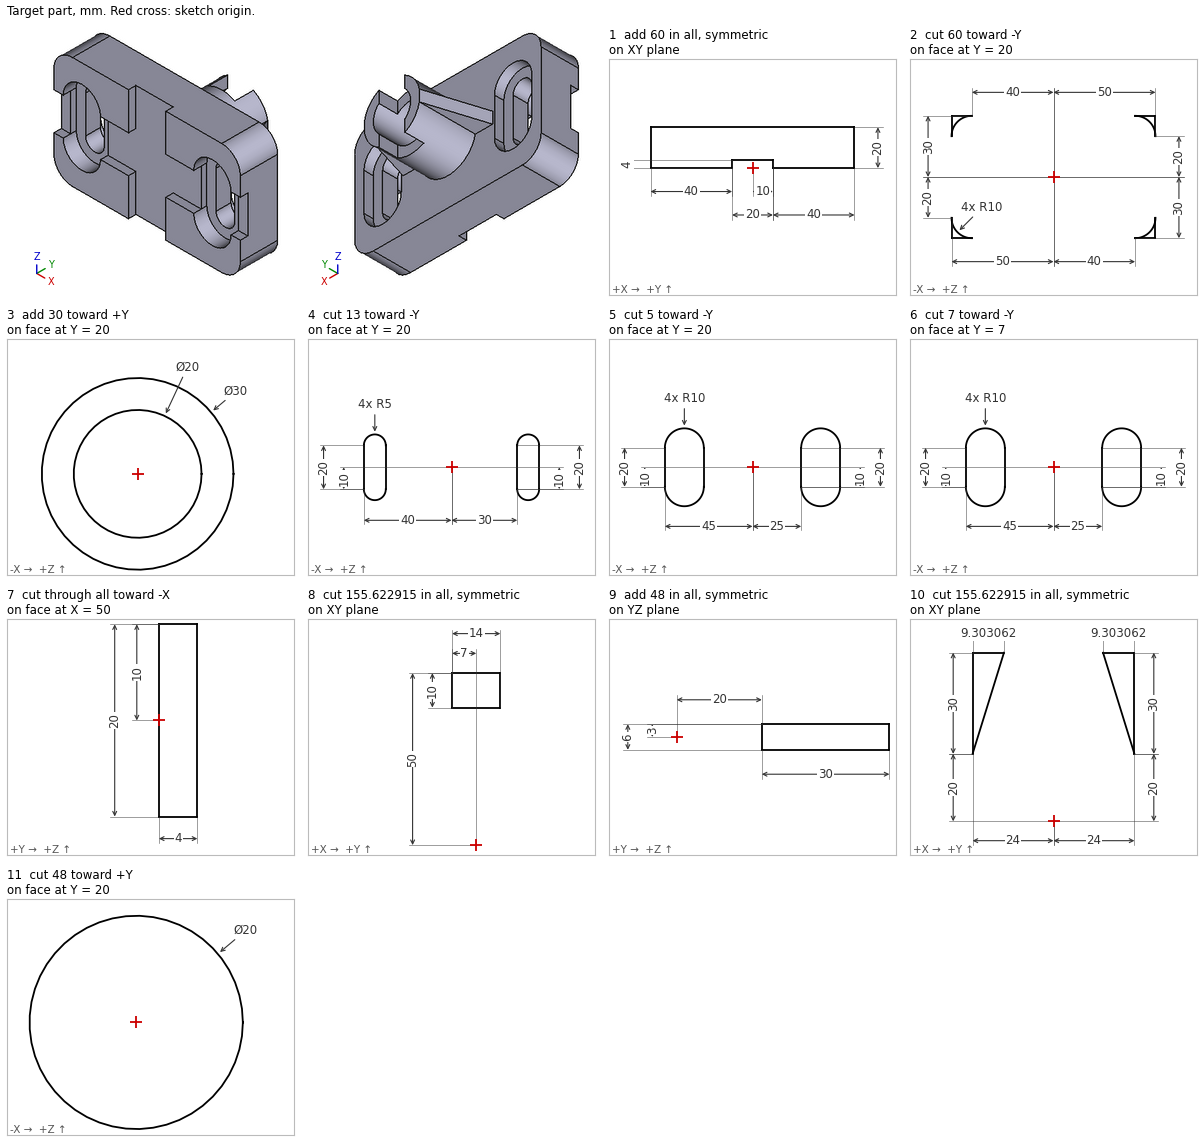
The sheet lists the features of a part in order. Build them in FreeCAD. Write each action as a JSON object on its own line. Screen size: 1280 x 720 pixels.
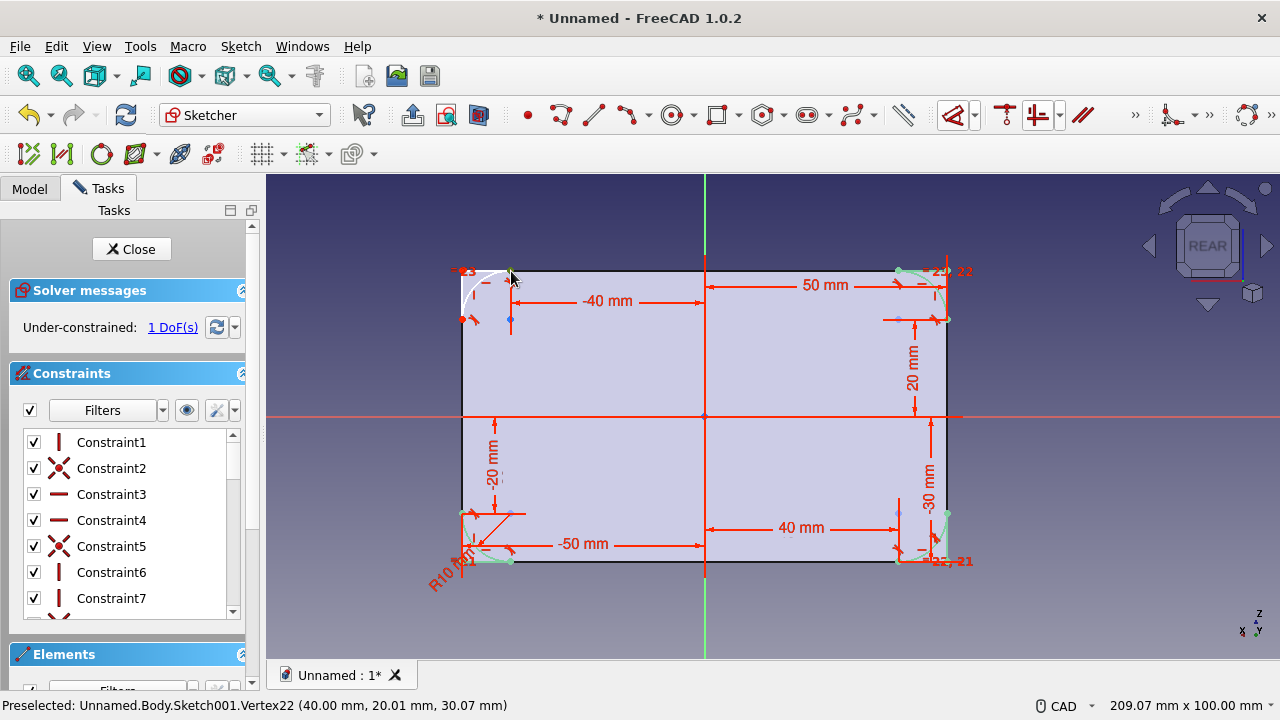
{"action": "left_click", "coordinate": [974, 116]}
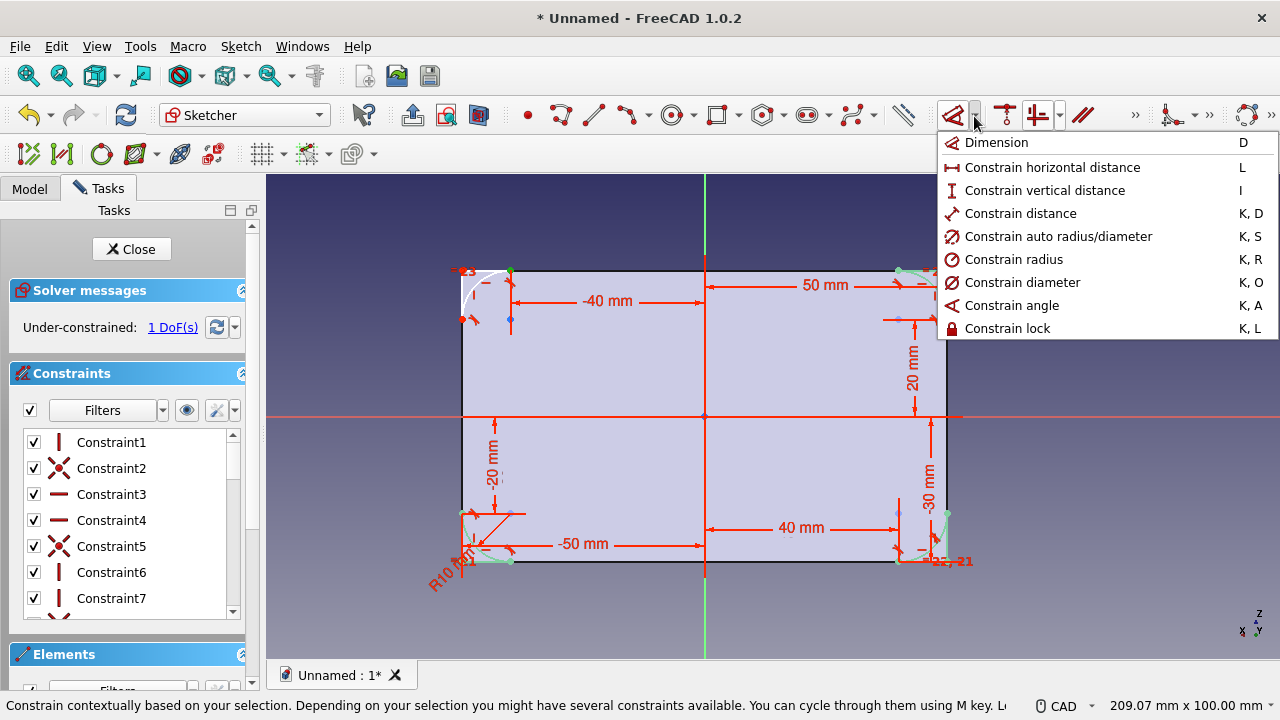
{"action": "left_click", "coordinate": [1108, 190]}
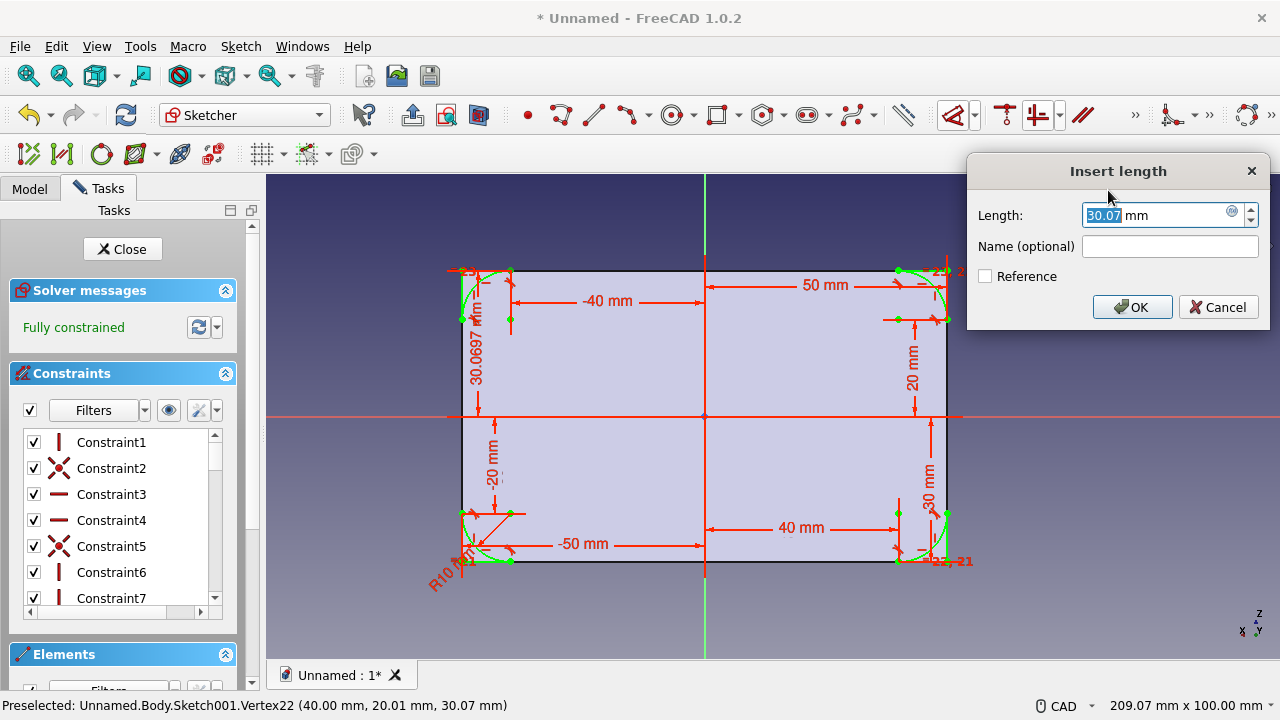
{"action": "type", "text": "30"}
{"action": "key", "text": "Return"}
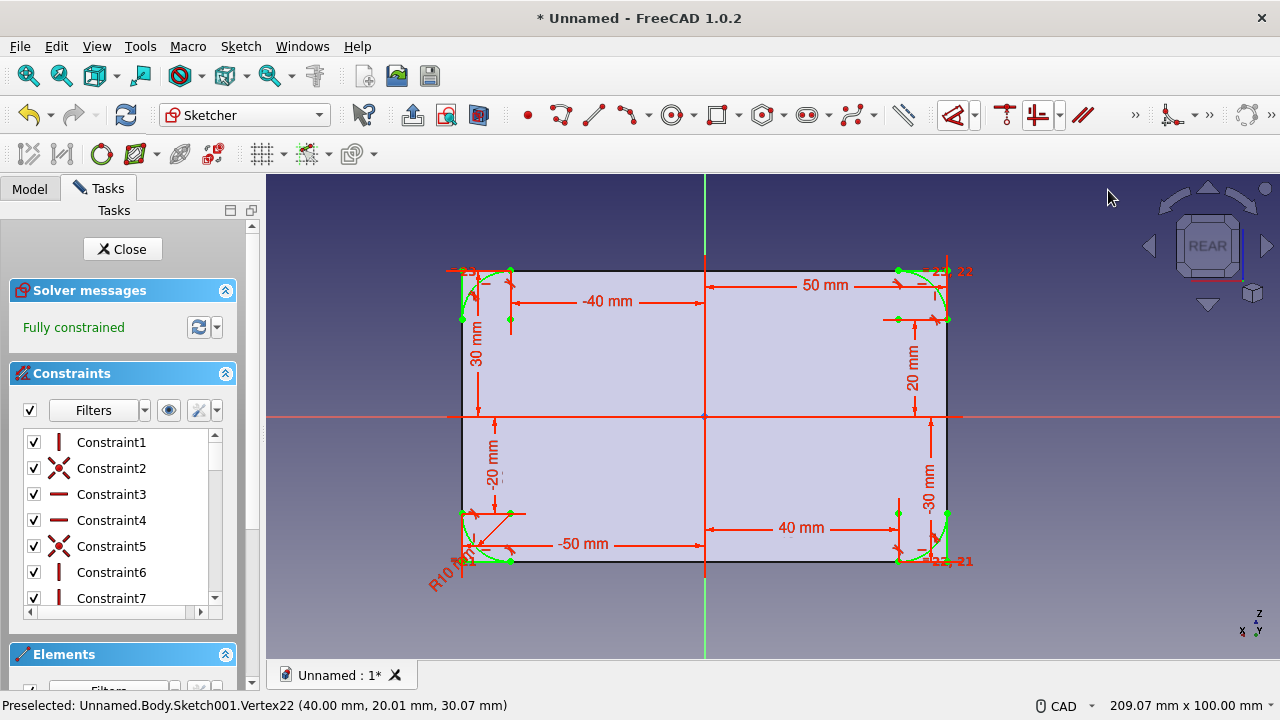
{"action": "left_click", "coordinate": [123, 249]}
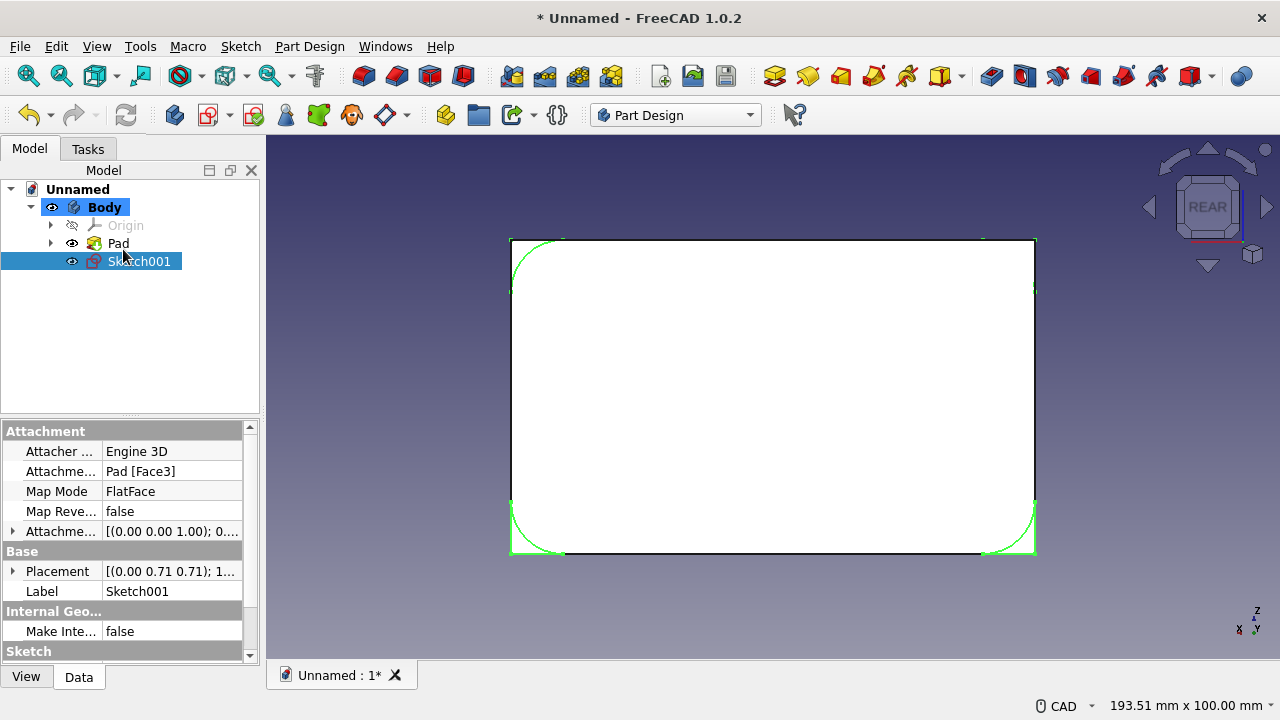
{"action": "left_click", "coordinate": [992, 76]}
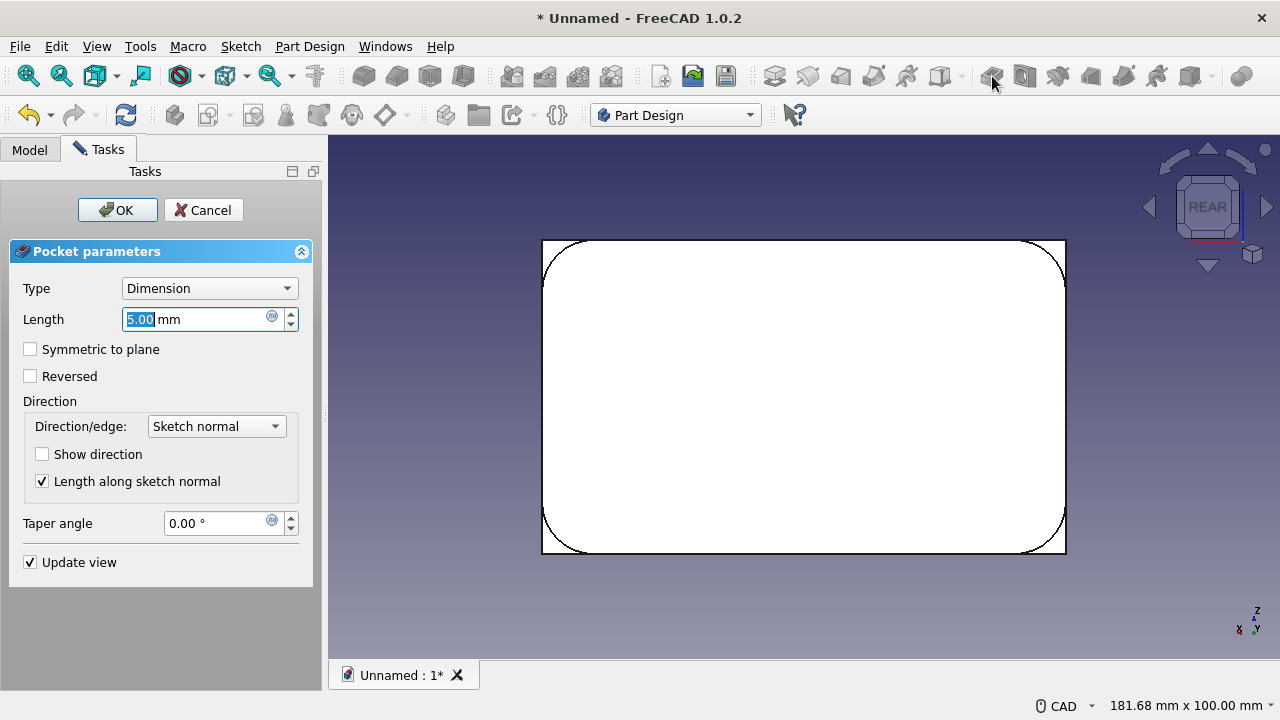
{"action": "type", "text": "60"}
{"action": "key", "text": "Tab"}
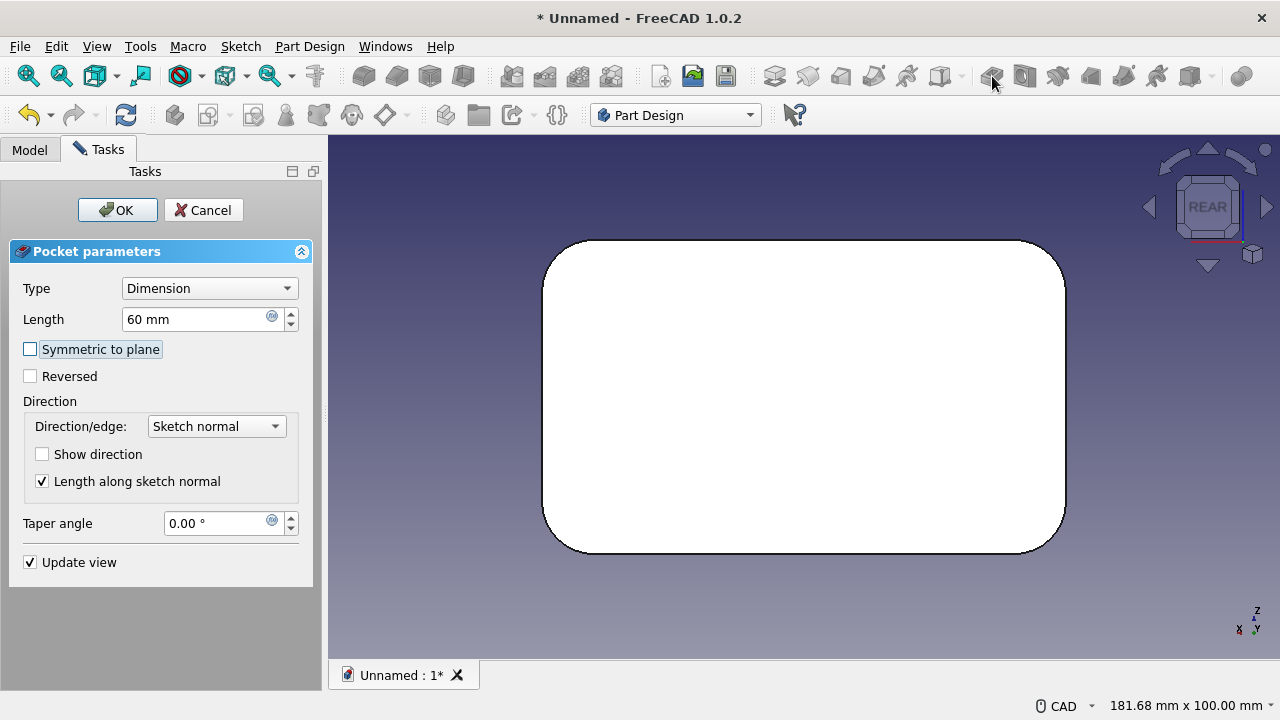
{"action": "left_click", "coordinate": [118, 210]}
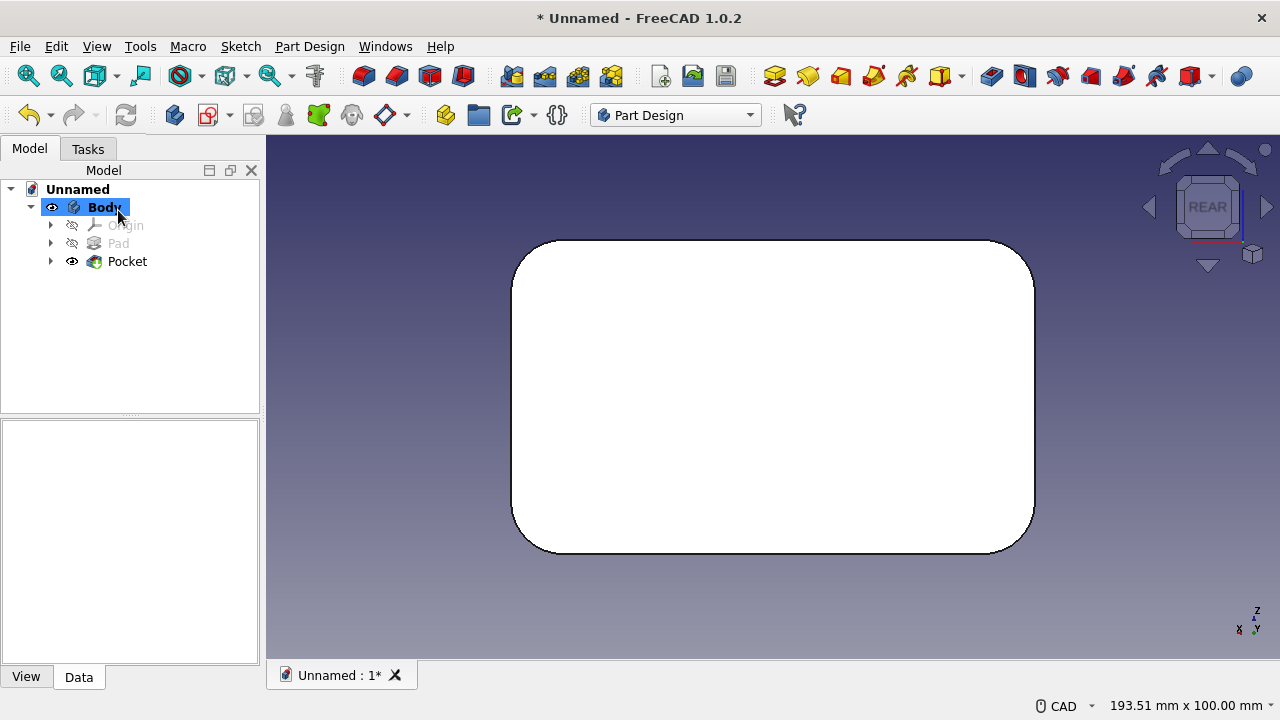
{"action": "left_click", "coordinate": [698, 396]}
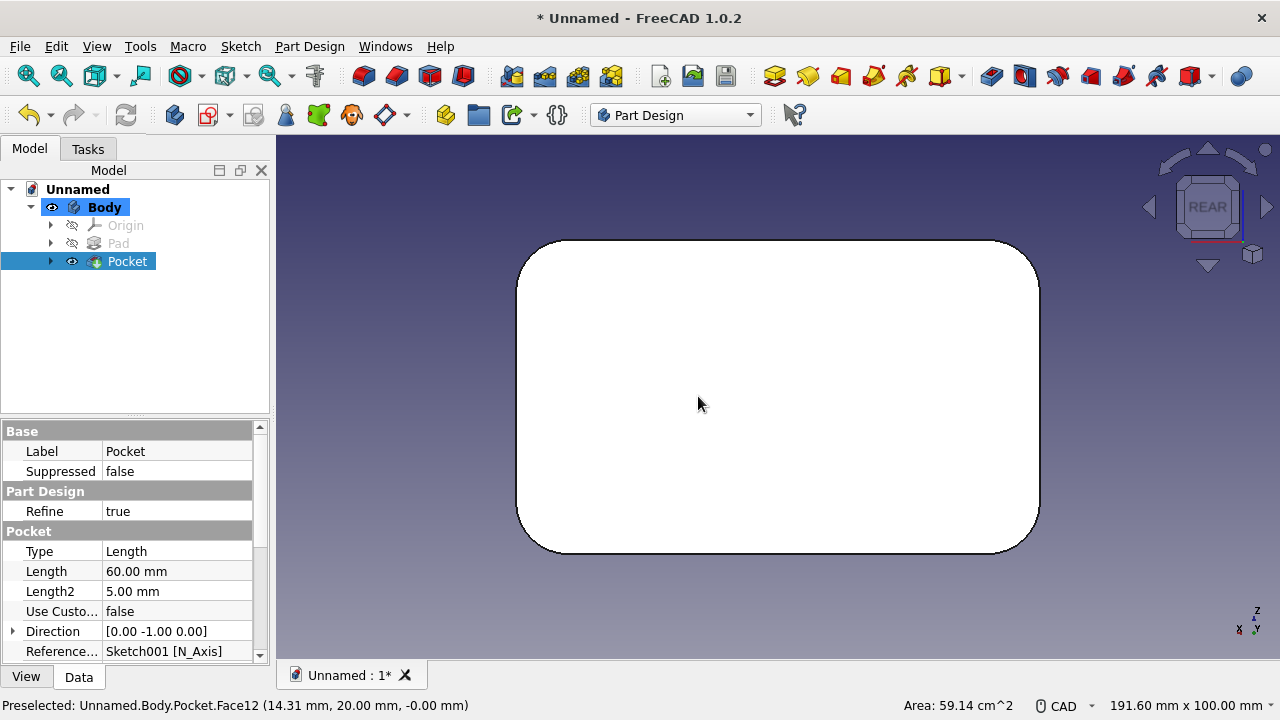
{"action": "left_click", "coordinate": [208, 116]}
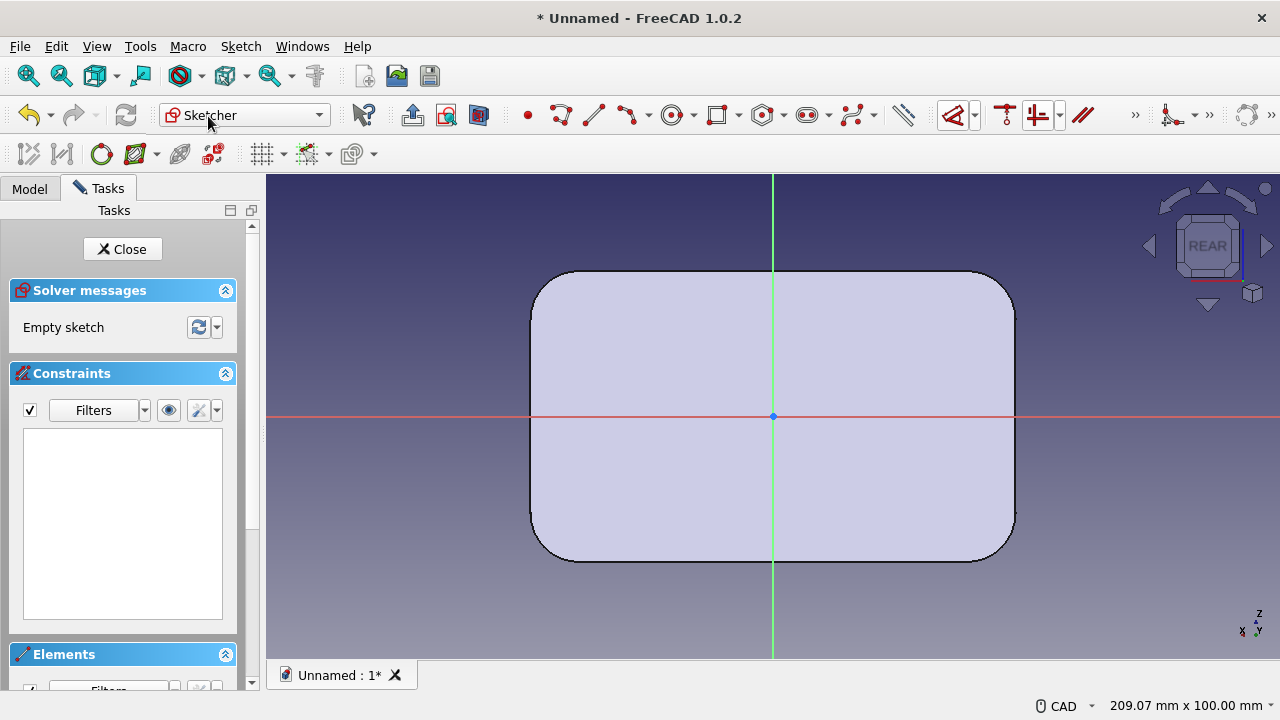
{"action": "scroll", "coordinate": [829, 417], "scroll_direction": "up", "scroll_amount": 4}